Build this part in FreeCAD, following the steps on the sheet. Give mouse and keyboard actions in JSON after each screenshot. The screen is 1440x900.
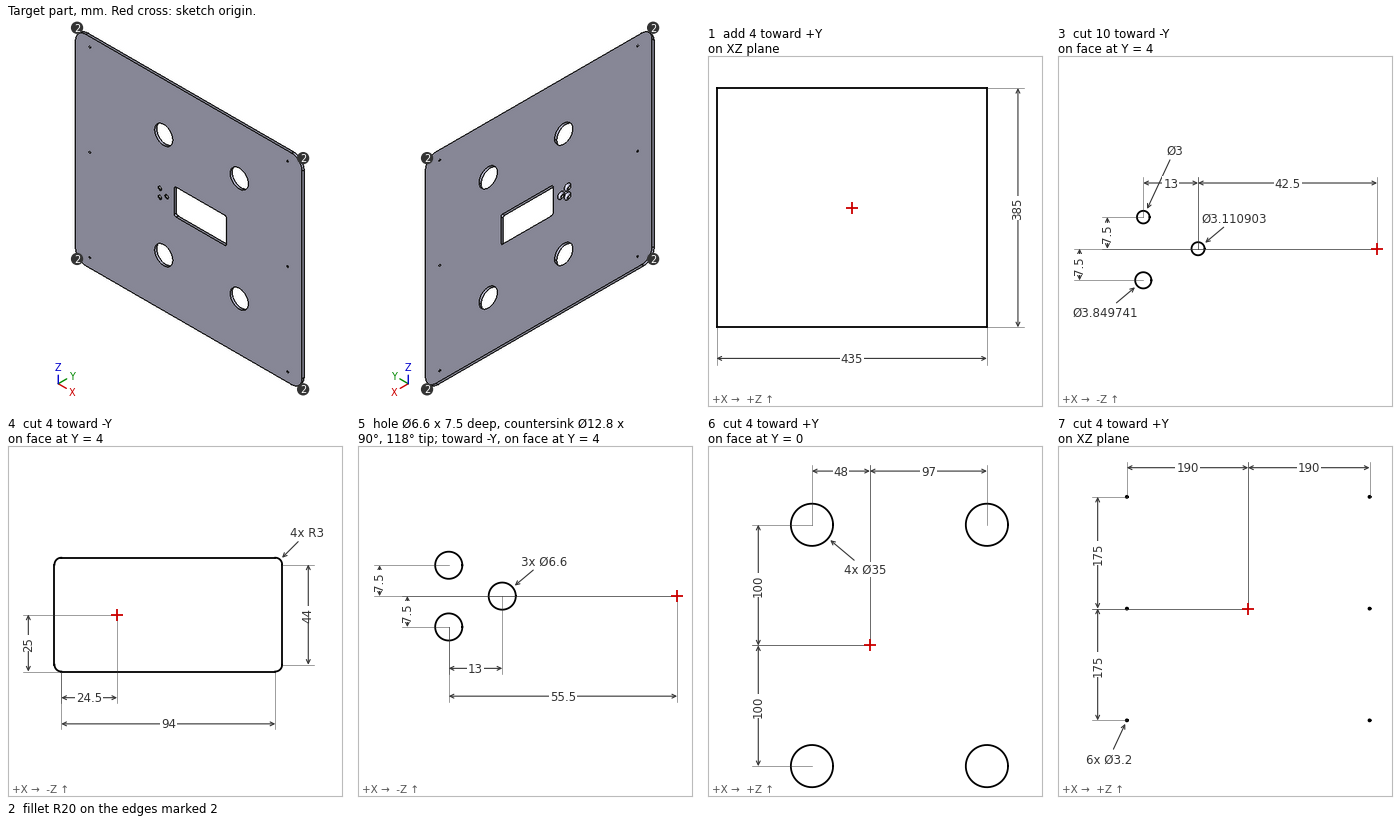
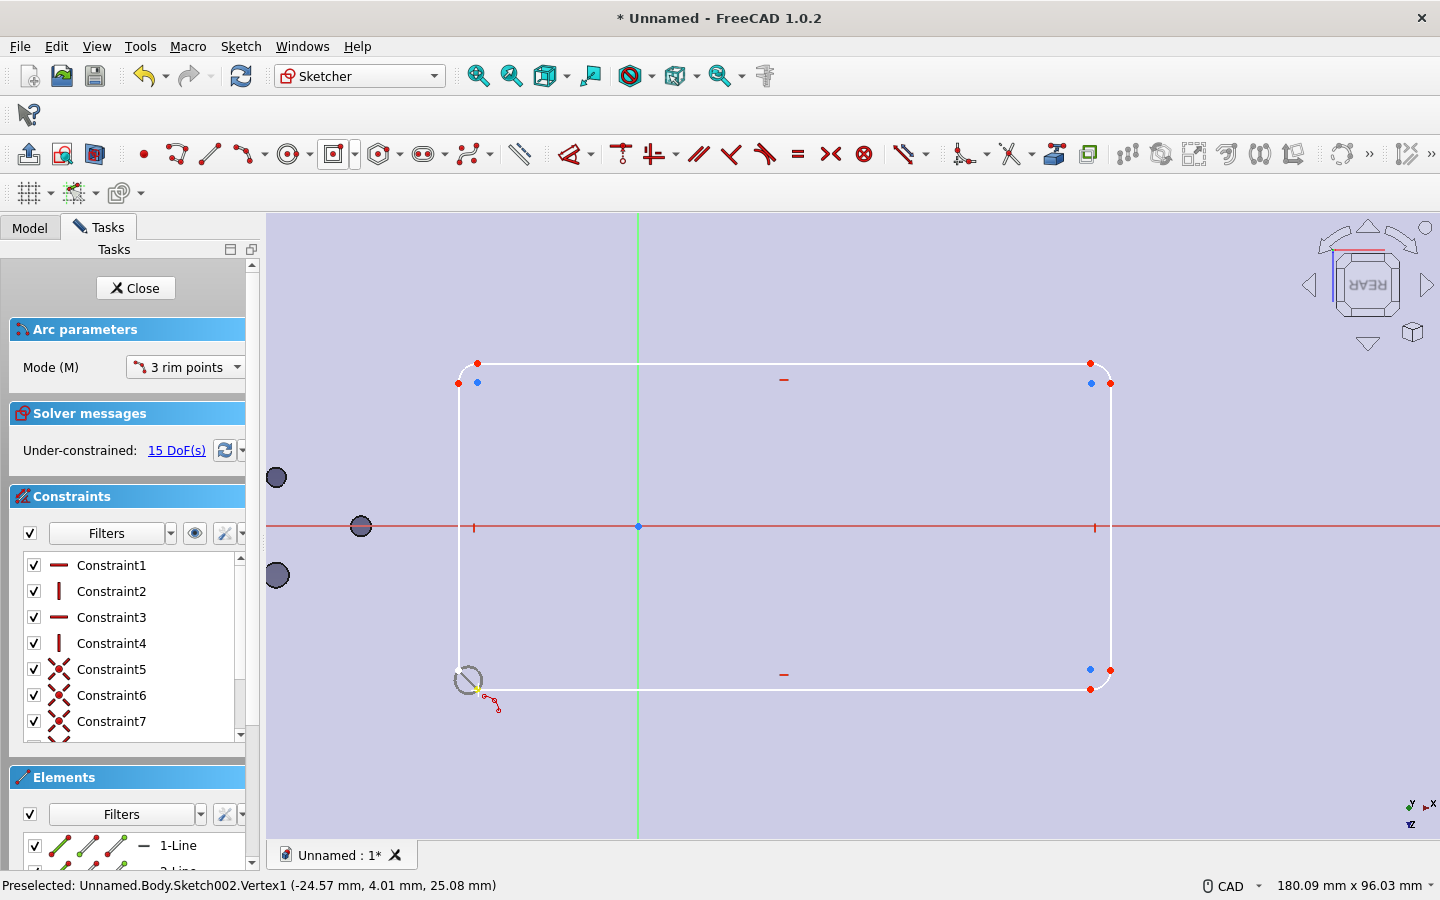
{"action": "scroll", "coordinate": [465, 684], "scroll_direction": "up", "scroll_amount": 6}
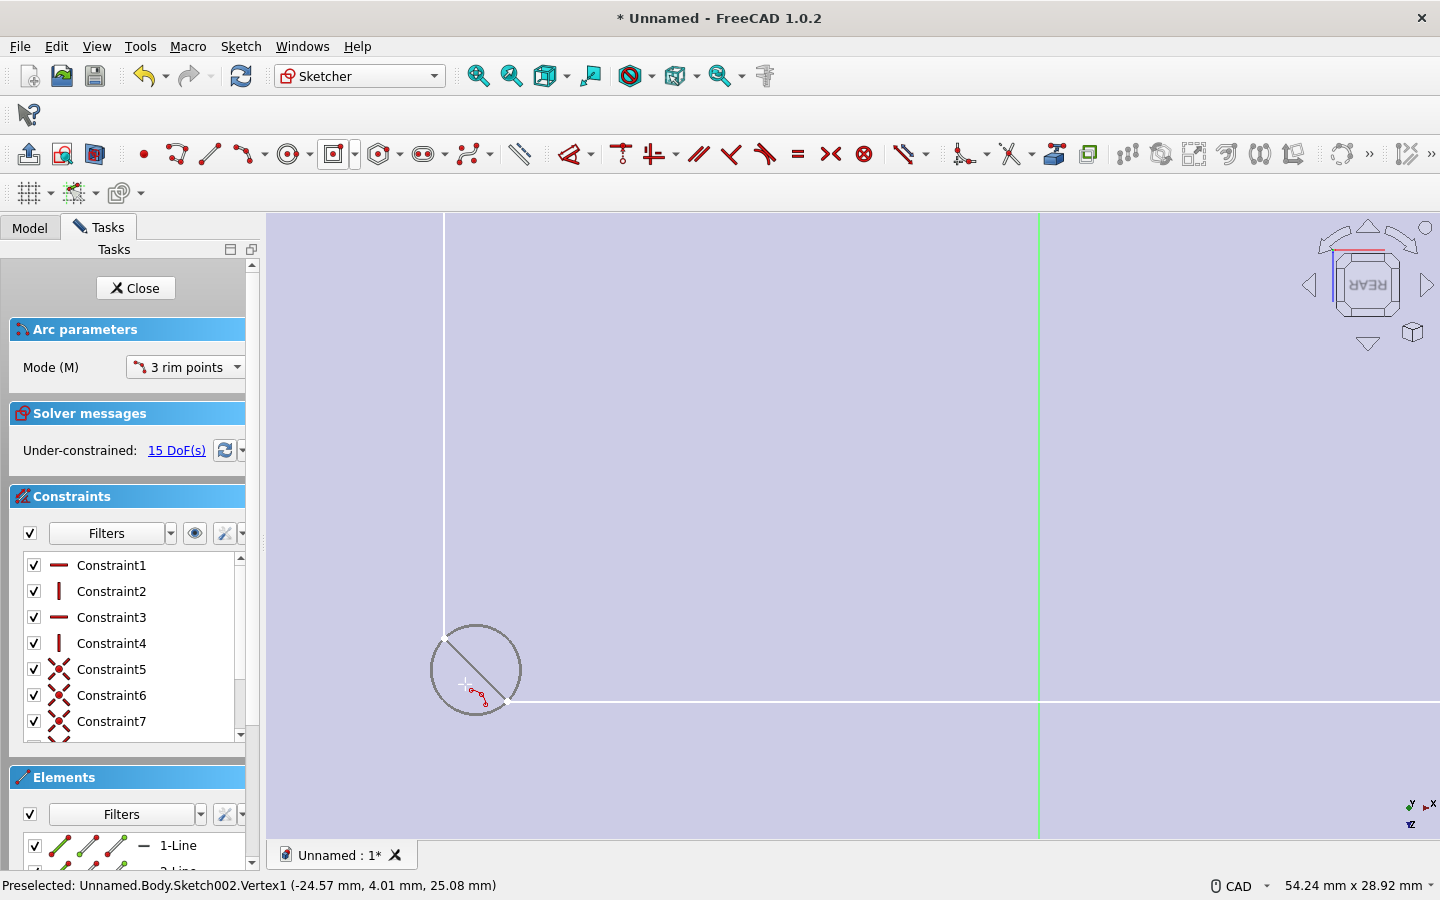
{"action": "left_click", "coordinate": [463, 681]}
{"action": "key", "text": "Escape"}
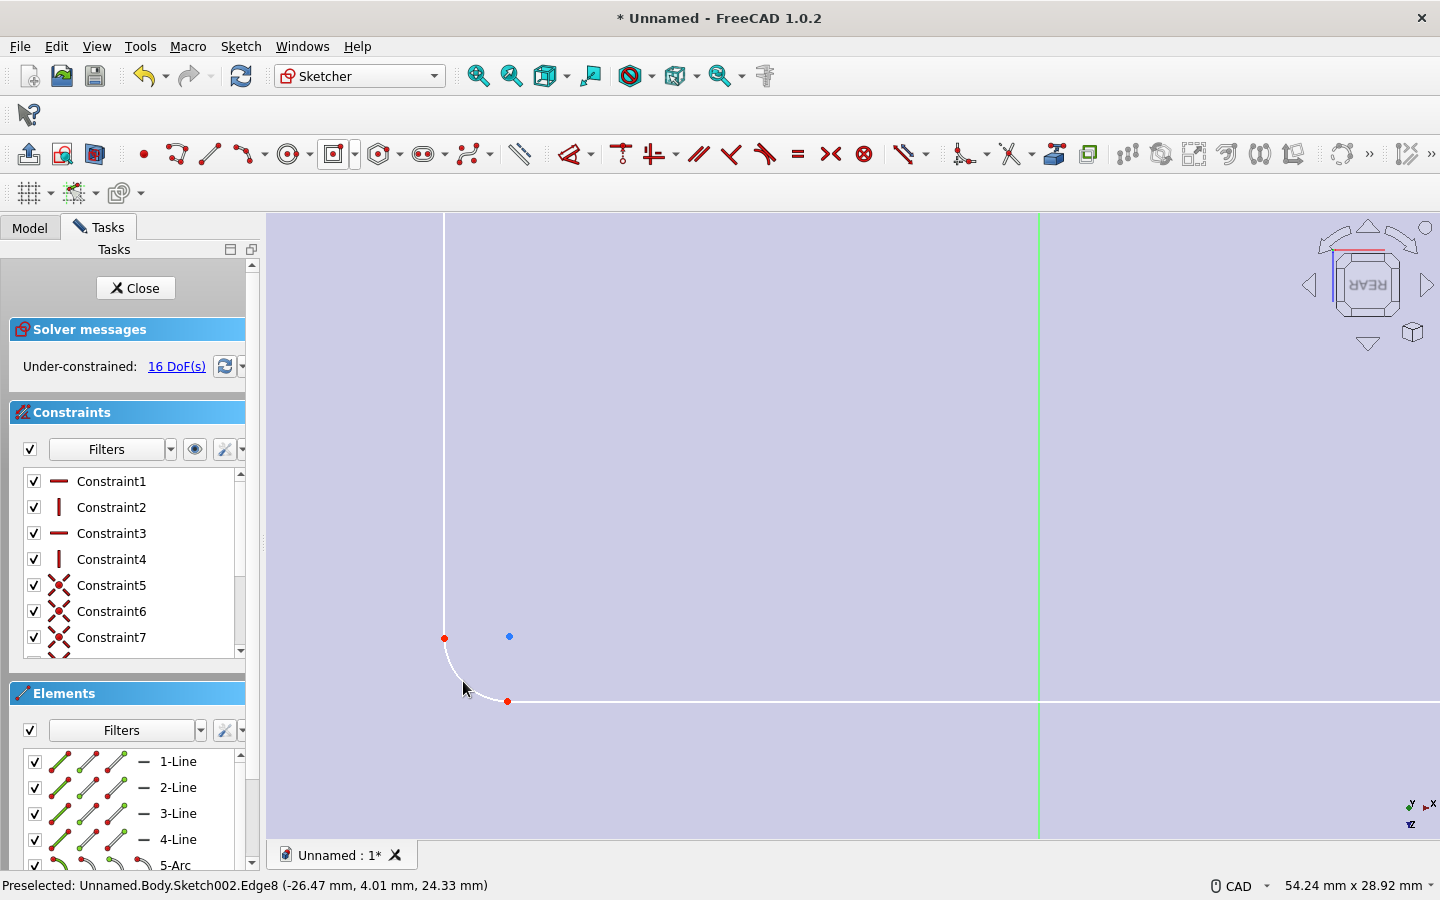
{"action": "left_click", "coordinate": [1118, 702]}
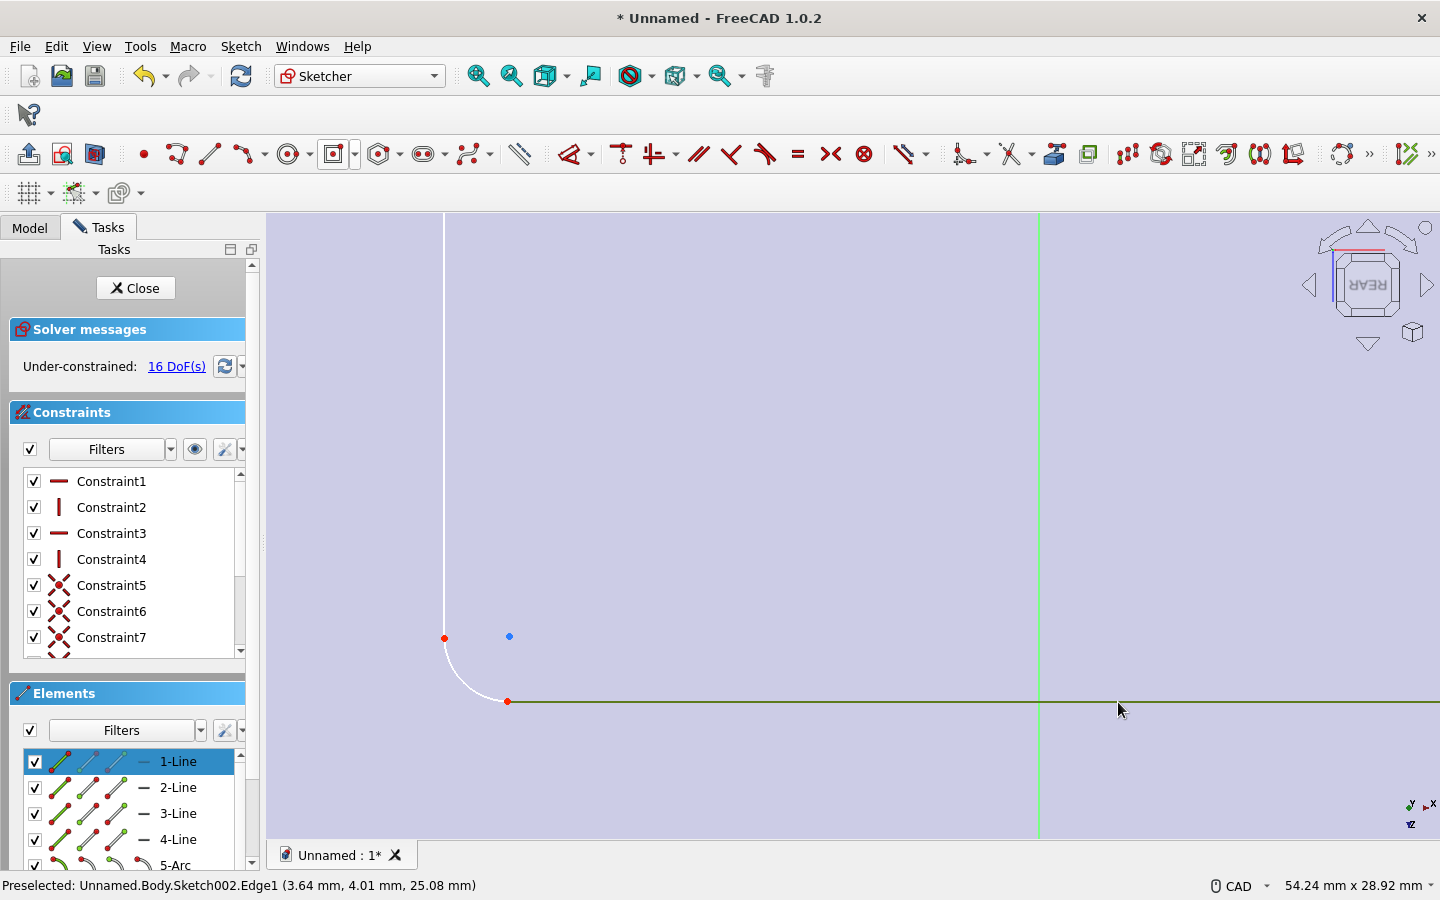
{"action": "scroll", "coordinate": [465, 684], "scroll_direction": "down", "scroll_amount": 6}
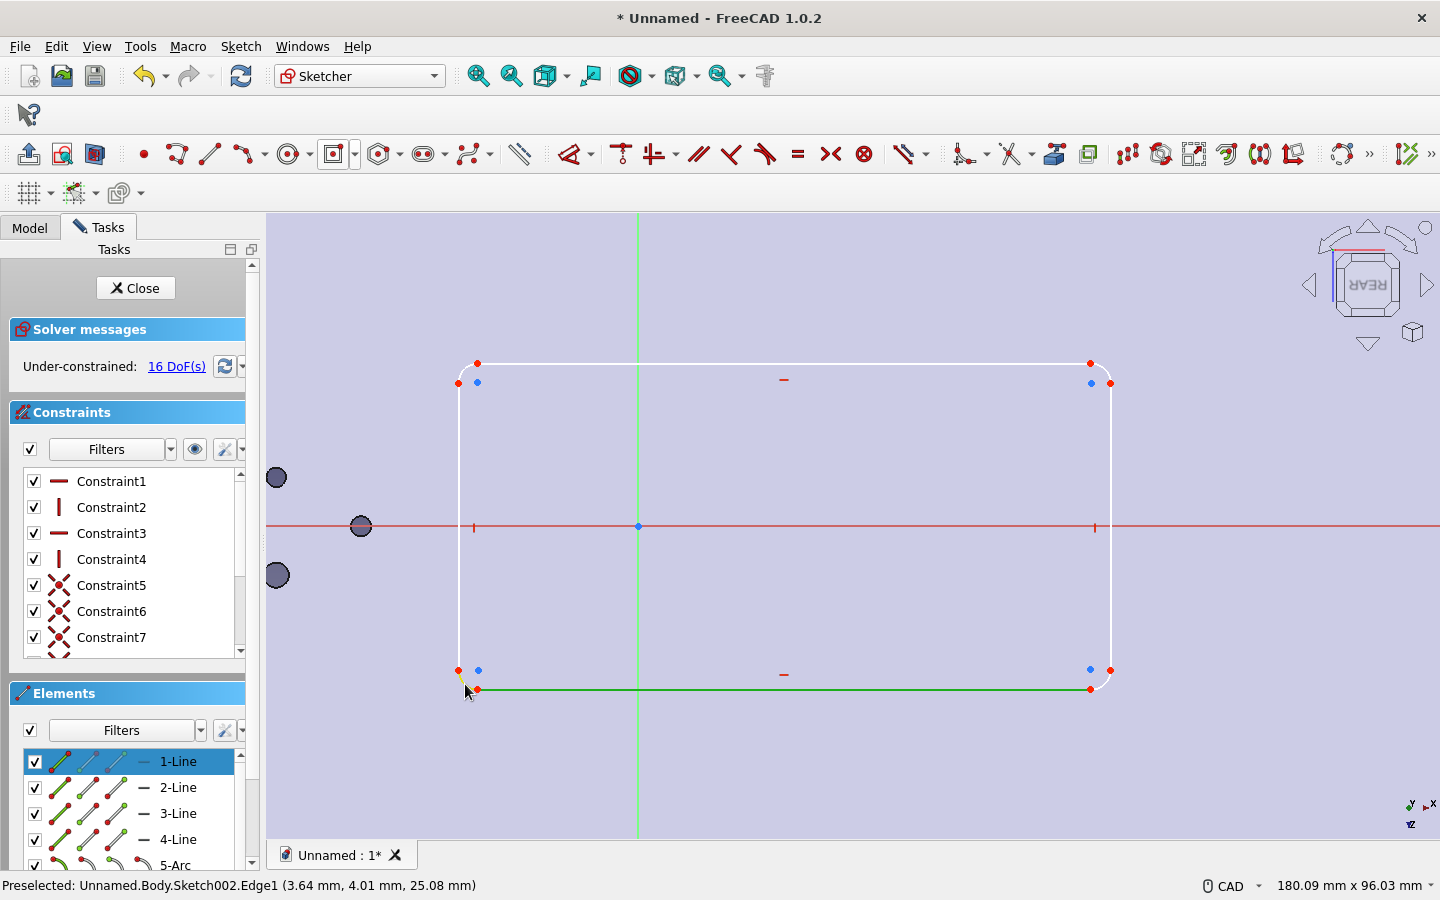
{"action": "scroll", "coordinate": [1100, 688], "scroll_direction": "up", "scroll_amount": 3}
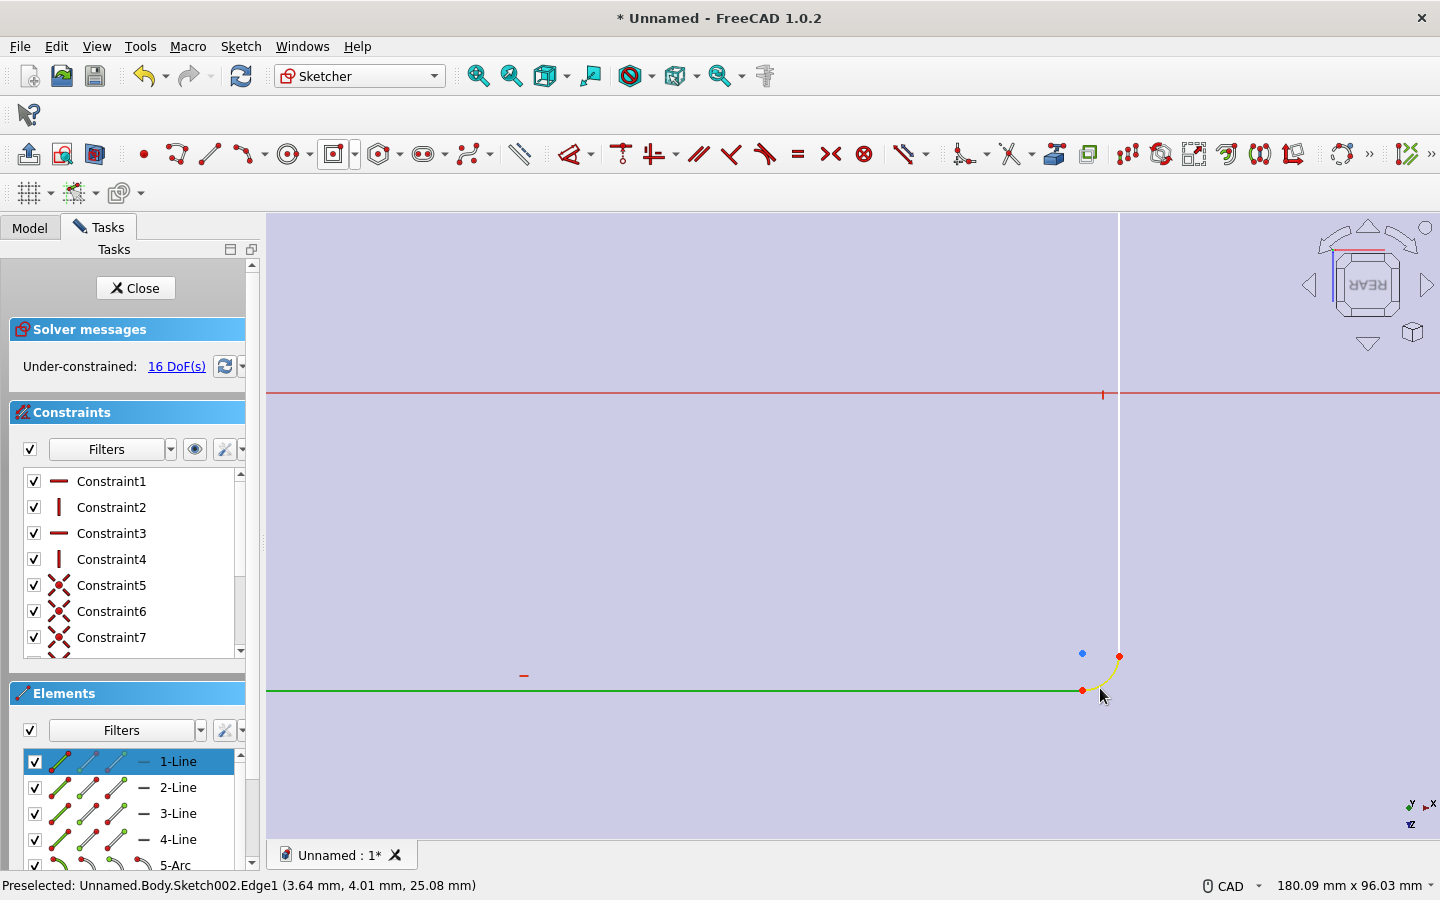
{"action": "left_click", "coordinate": [1099, 687]}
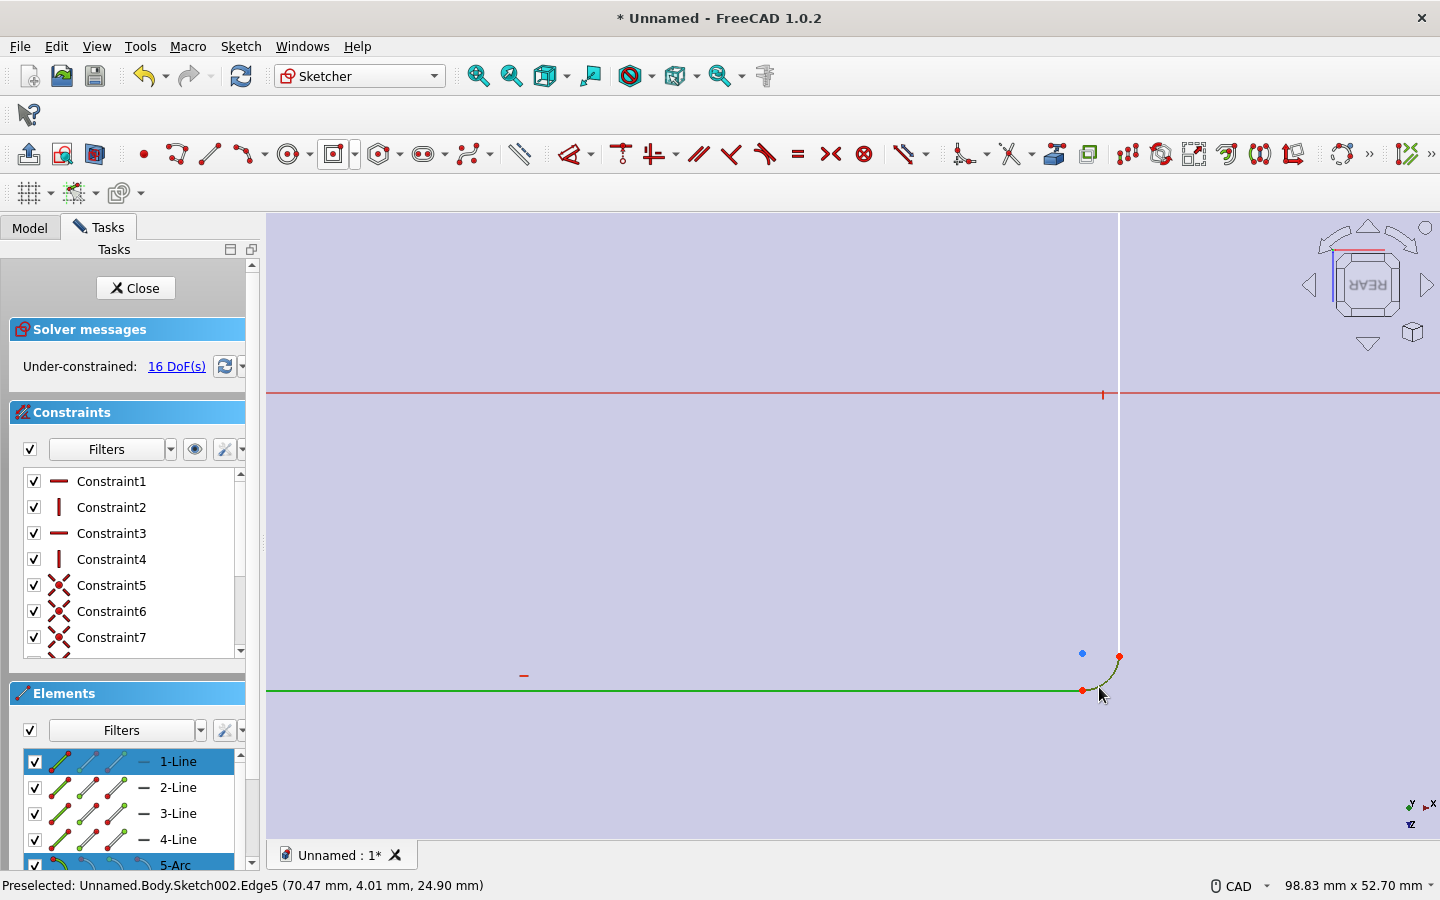
{"action": "left_click", "coordinate": [765, 154]}